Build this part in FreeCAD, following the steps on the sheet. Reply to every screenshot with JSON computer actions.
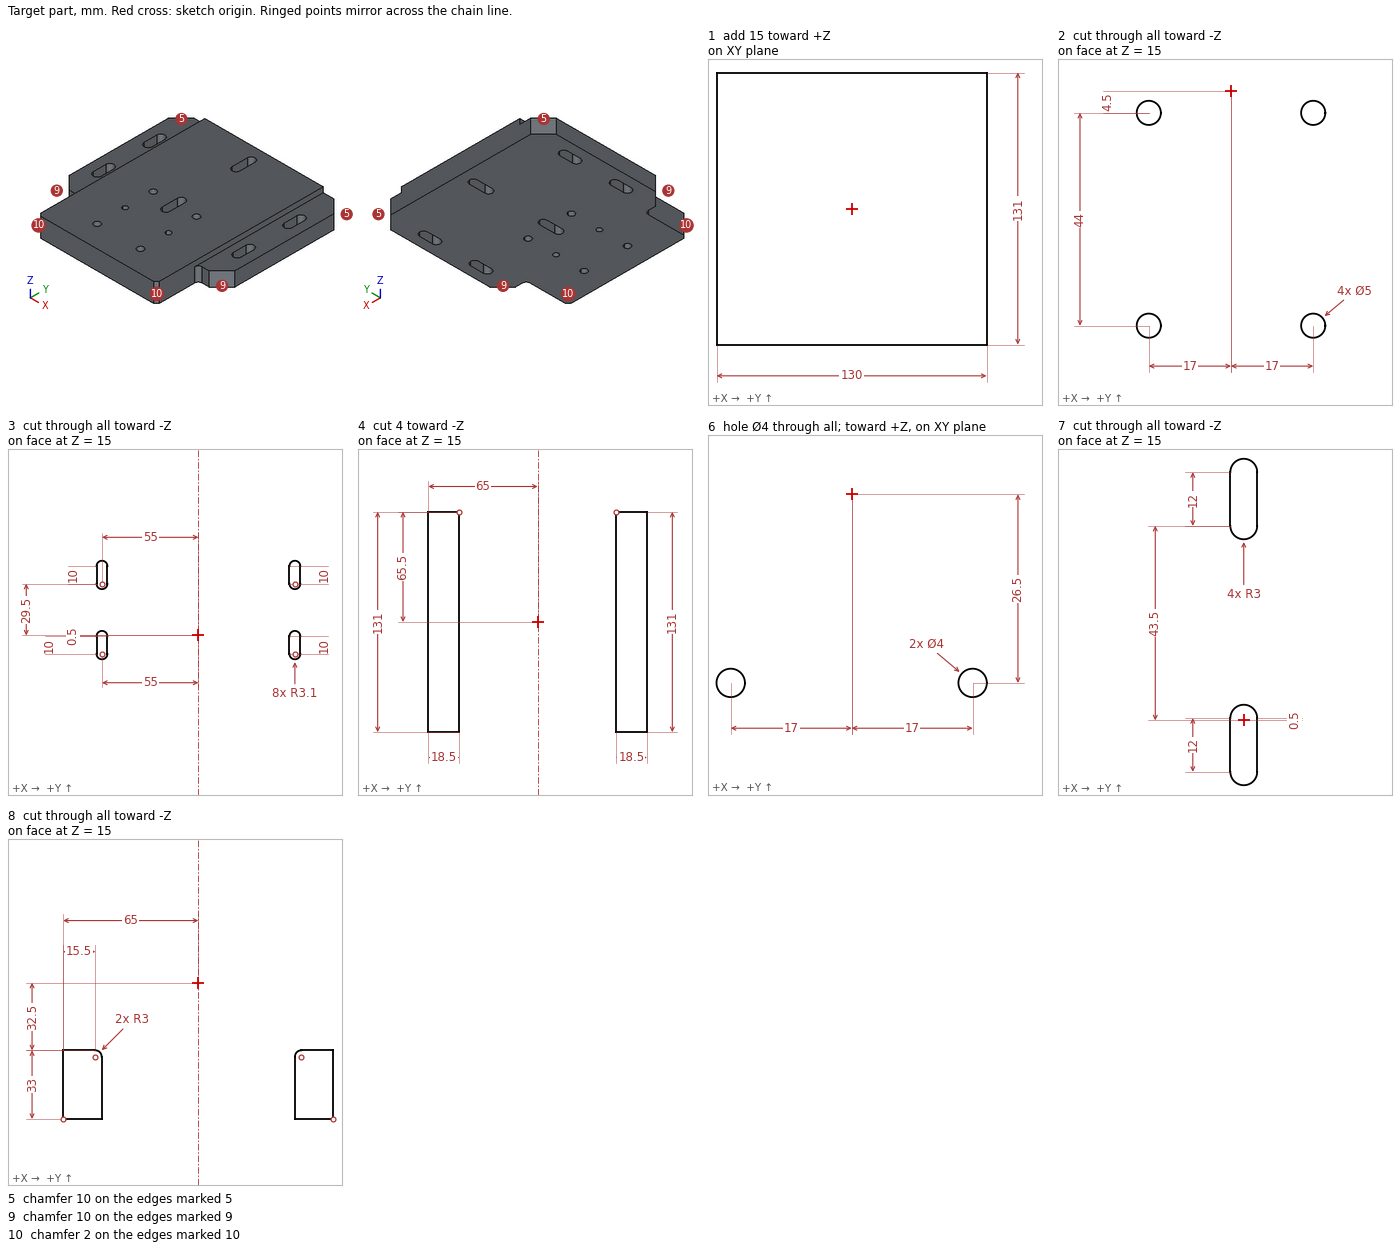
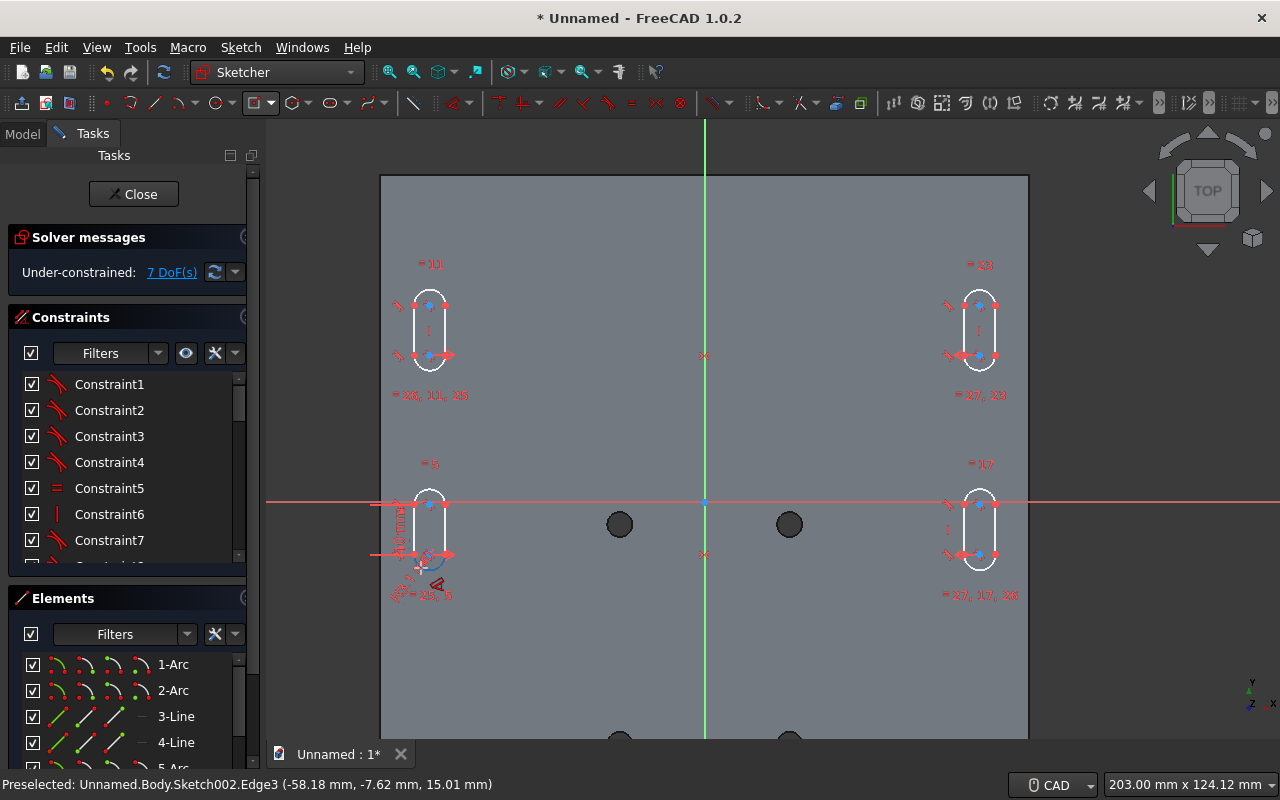
{"action": "left_click", "coordinate": [414, 340]}
{"action": "left_click", "coordinate": [380, 330]}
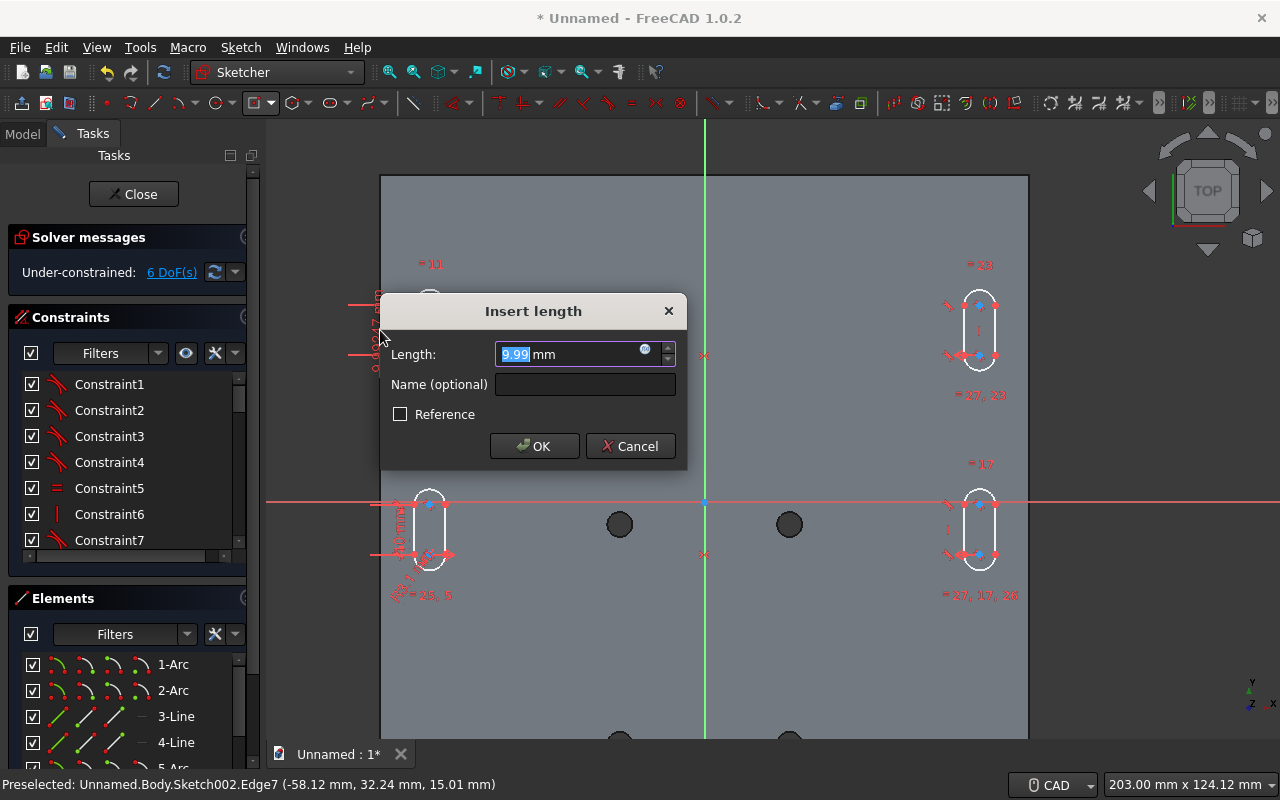
{"action": "type", "text": "10"}
{"action": "key", "text": "Return"}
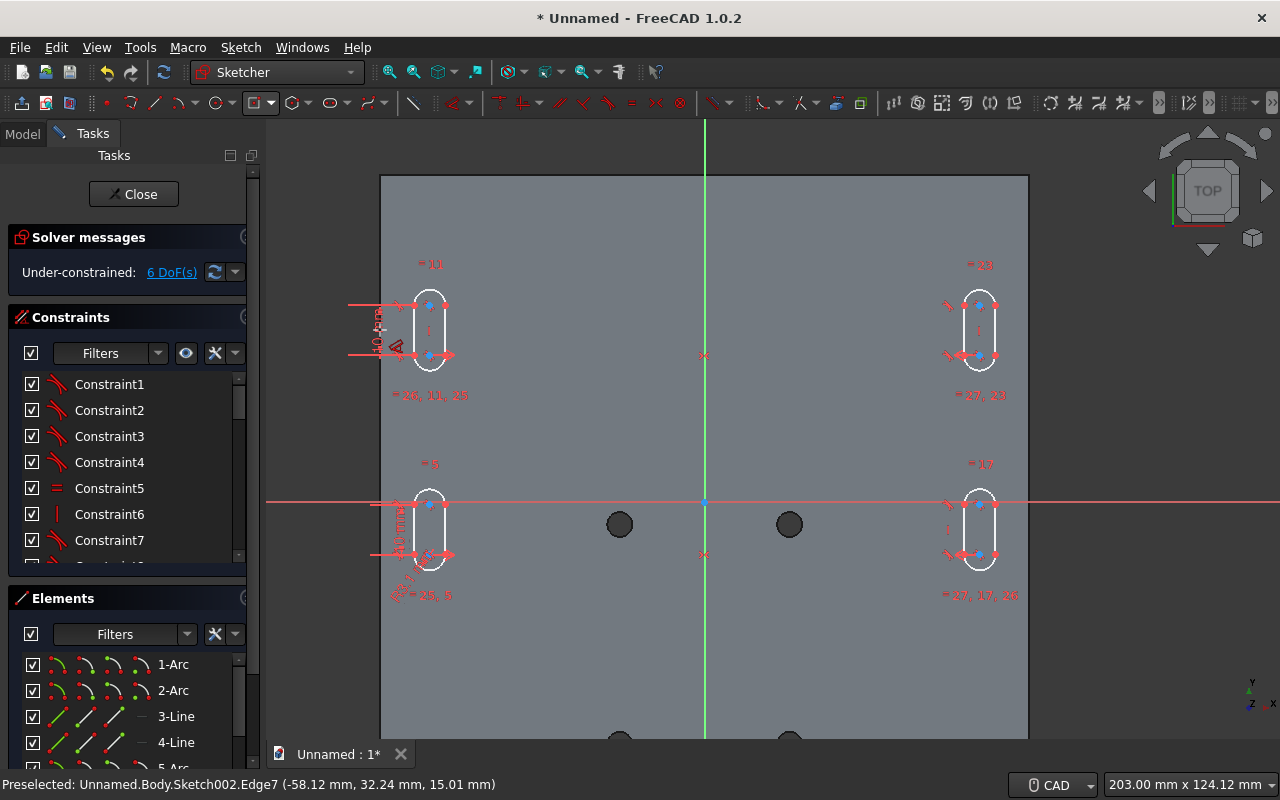
{"action": "left_click", "coordinate": [964, 540]}
{"action": "left_click", "coordinate": [930, 530]}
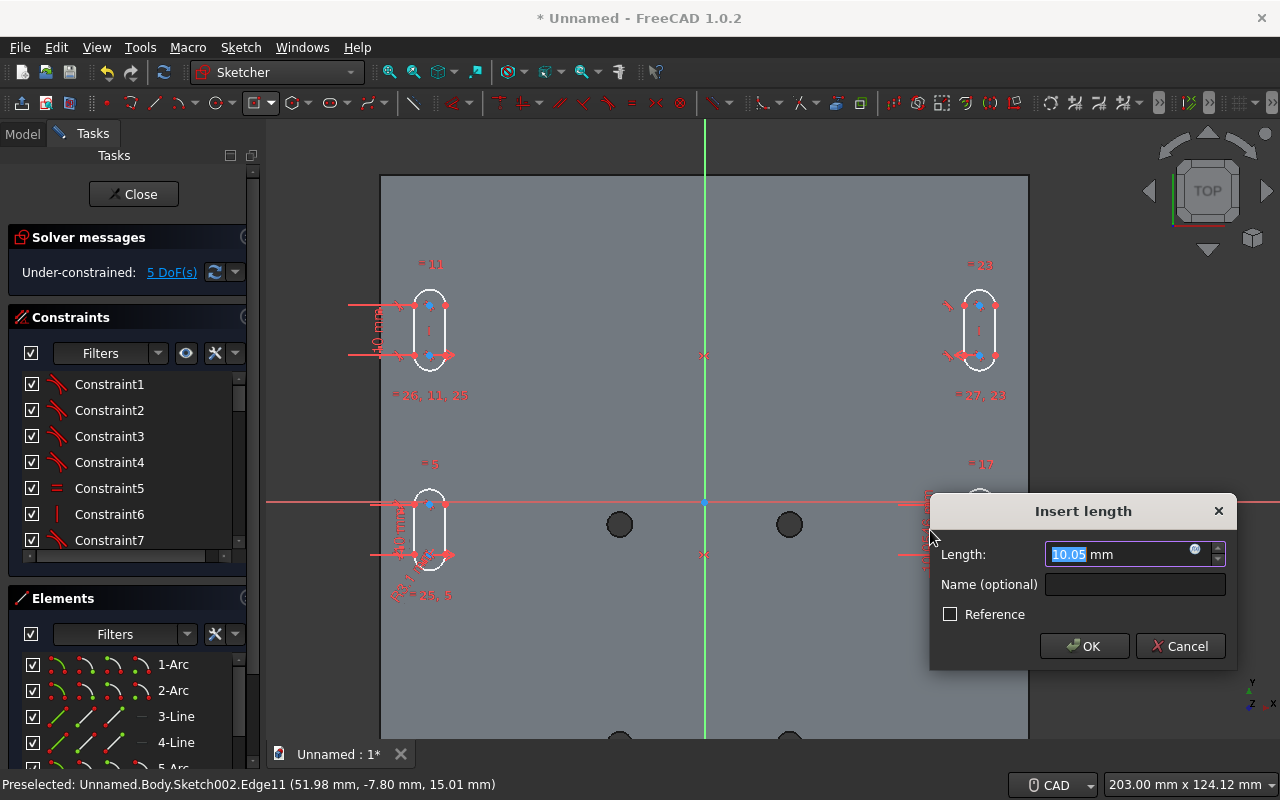
{"action": "type", "text": "10"}
{"action": "key", "text": "Return"}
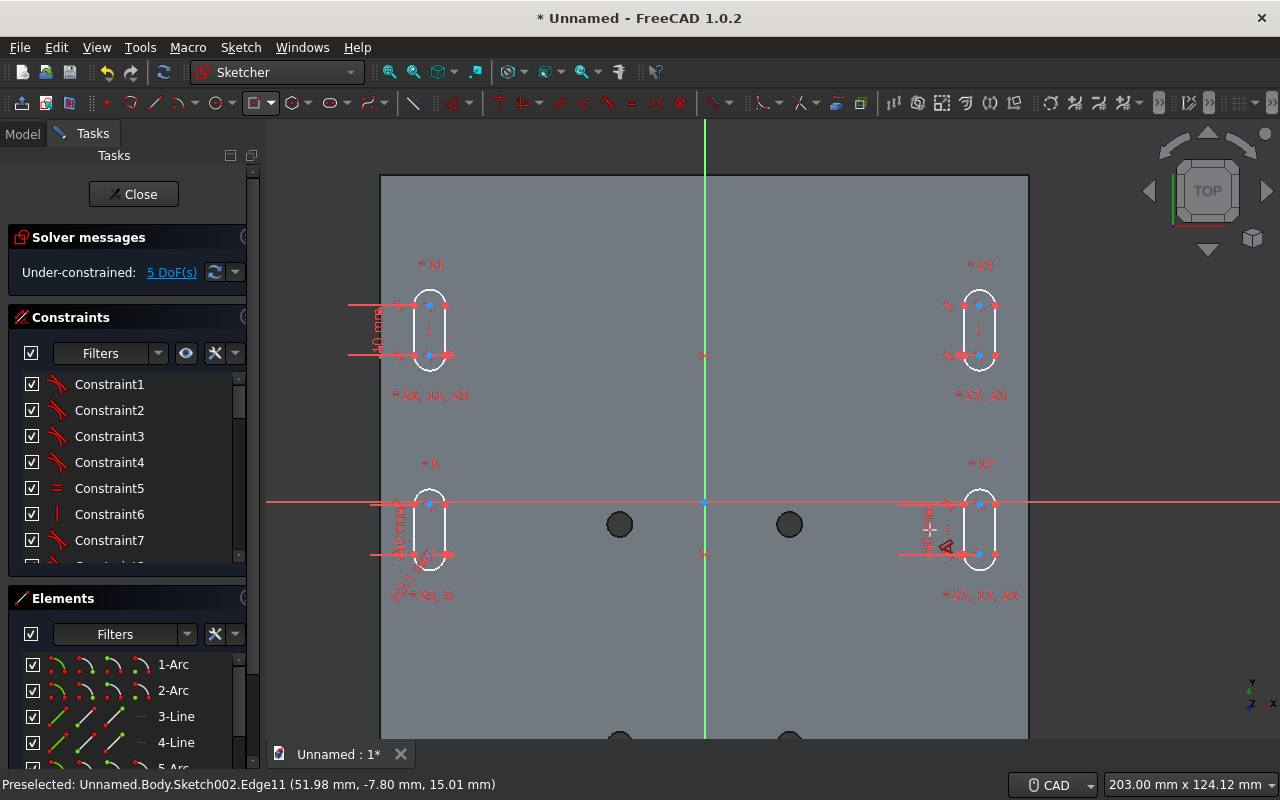
{"action": "left_click", "coordinate": [964, 340]}
{"action": "left_click", "coordinate": [930, 330]}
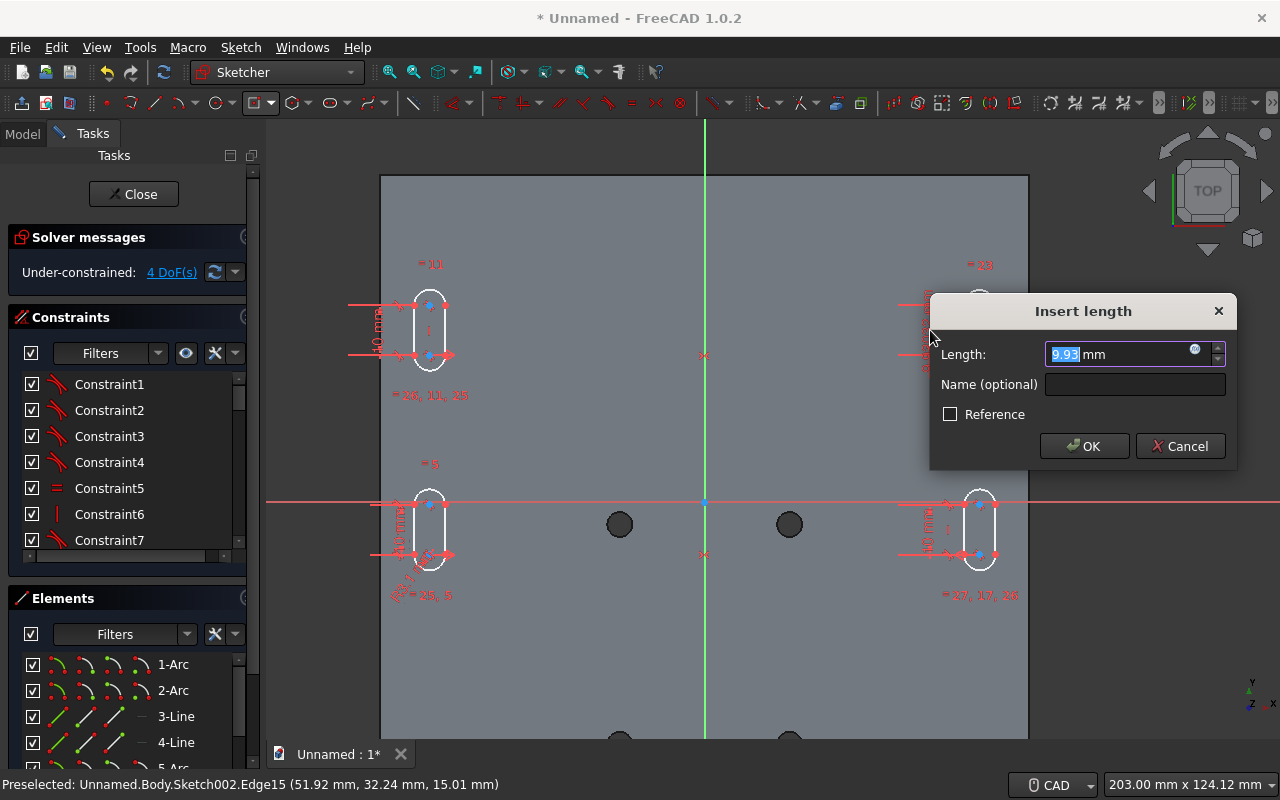
{"action": "type", "text": "10"}
{"action": "key", "text": "Return"}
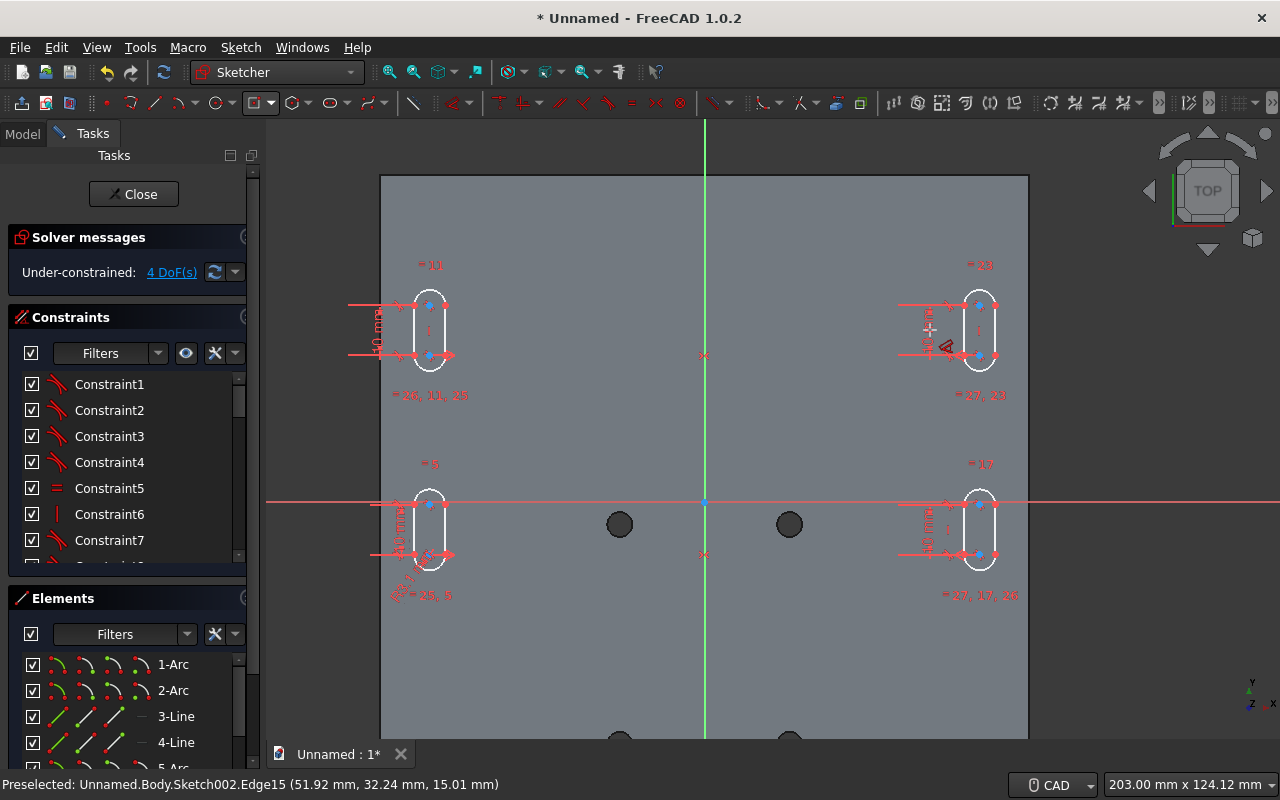
{"action": "left_click", "coordinate": [430, 555]}
{"action": "left_click", "coordinate": [567, 589]}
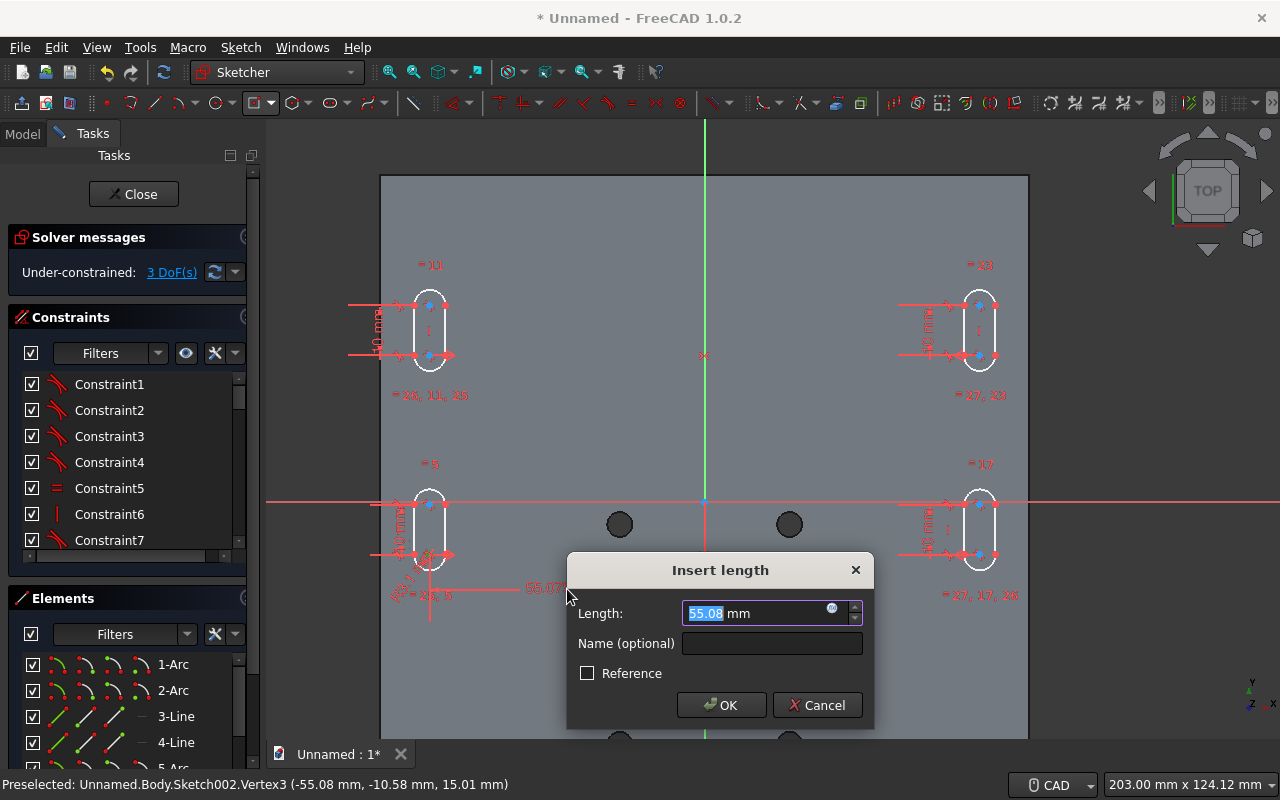
{"action": "type", "text": "55"}
{"action": "key", "text": "Return"}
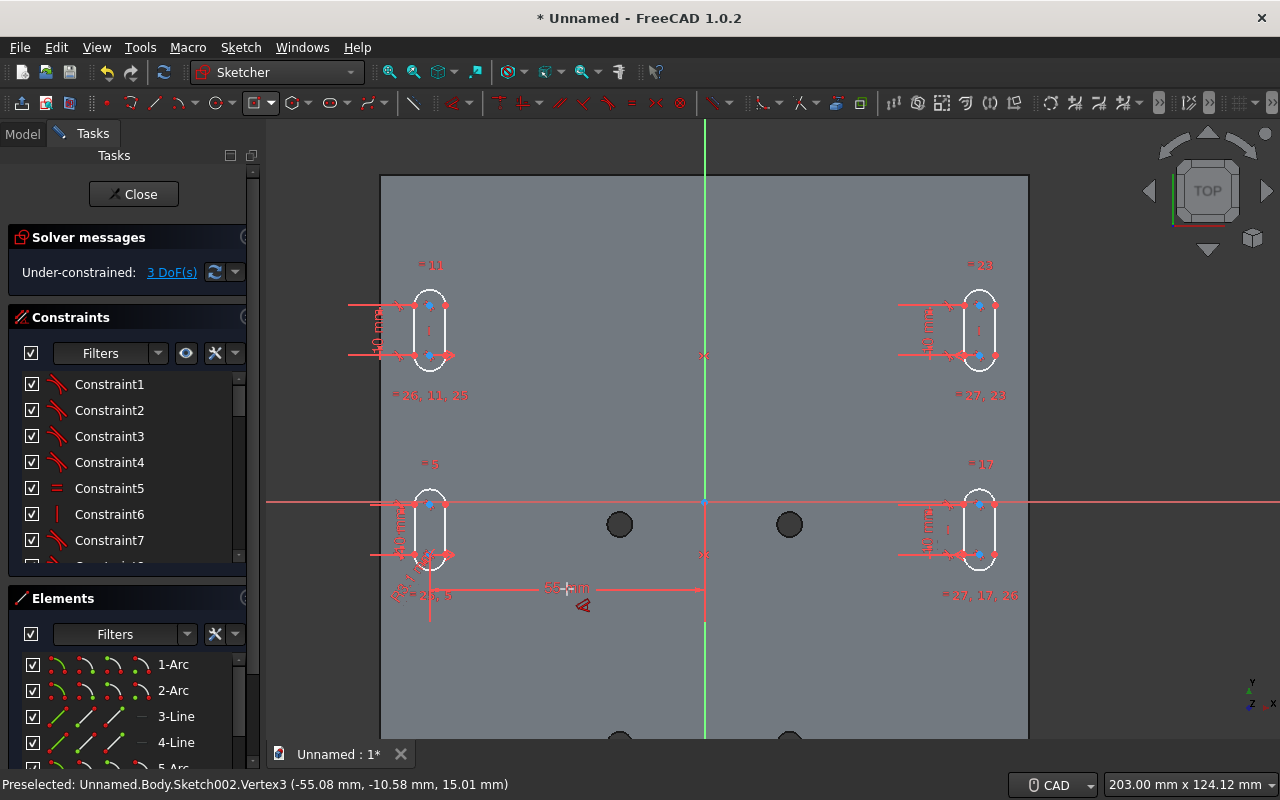
{"action": "left_click", "coordinate": [430, 355]}
{"action": "left_click", "coordinate": [567, 321]}